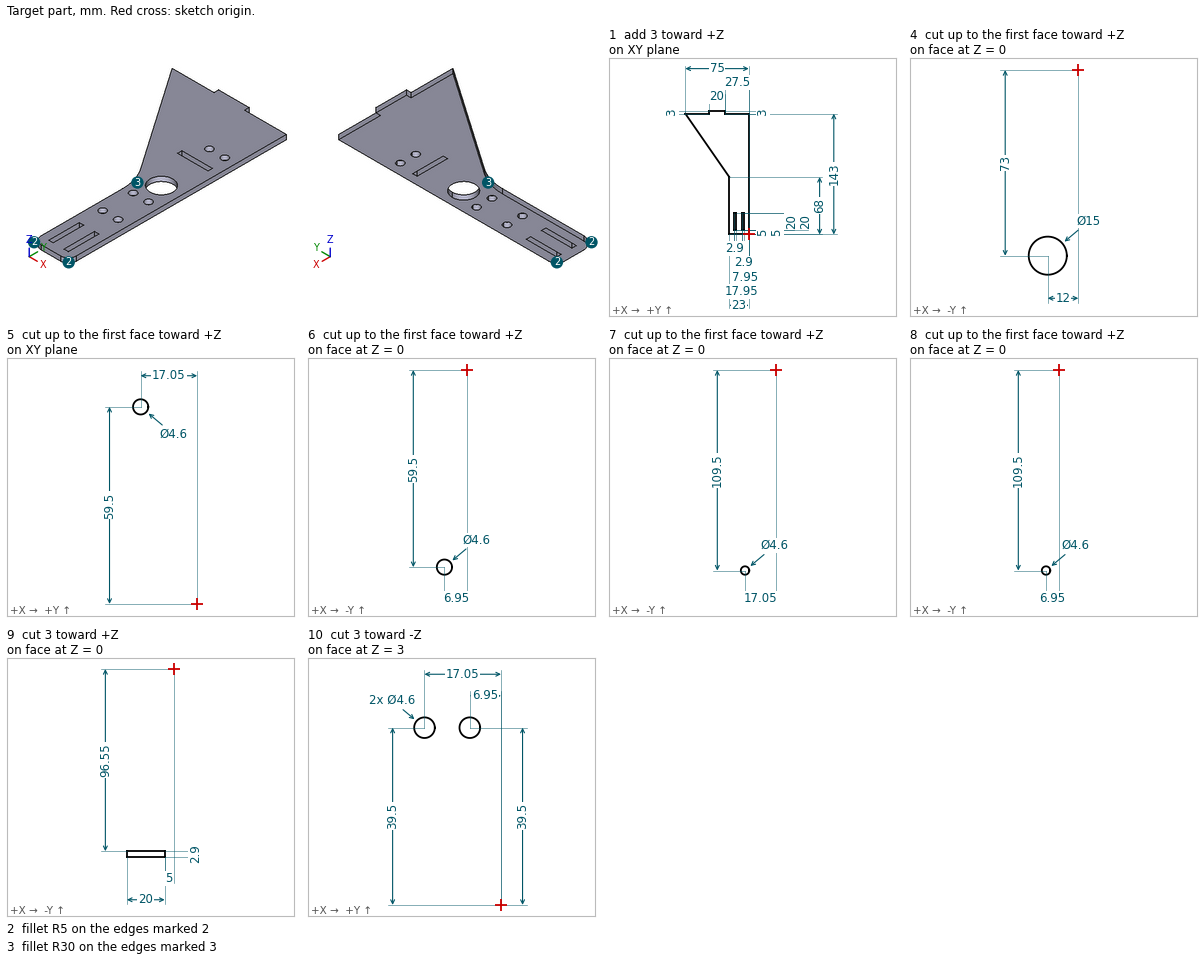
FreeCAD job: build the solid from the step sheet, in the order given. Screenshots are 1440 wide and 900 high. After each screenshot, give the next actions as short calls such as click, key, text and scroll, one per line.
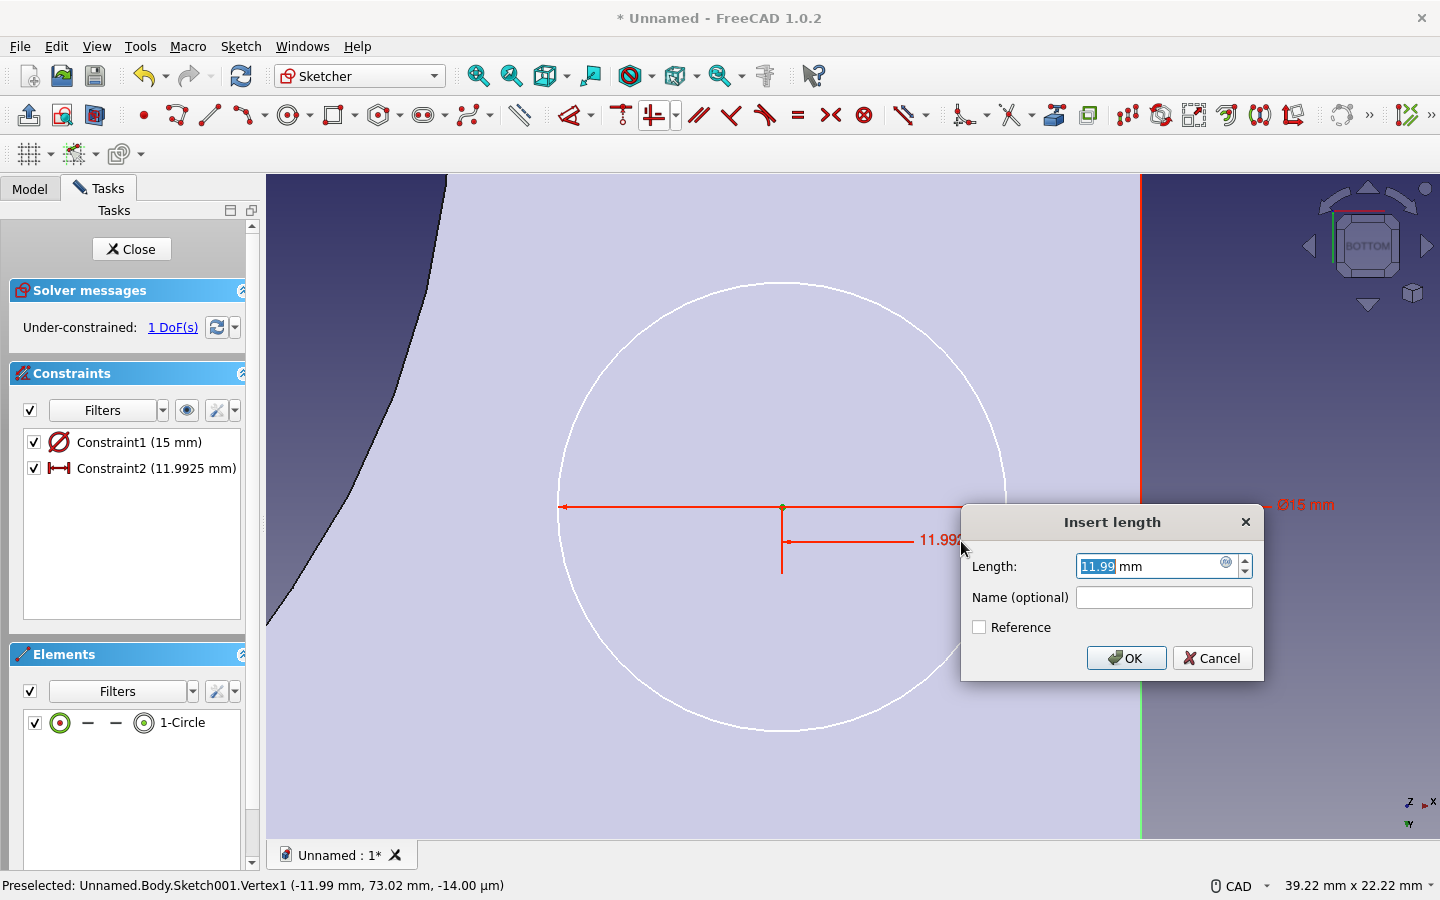
text(12)
key(Return)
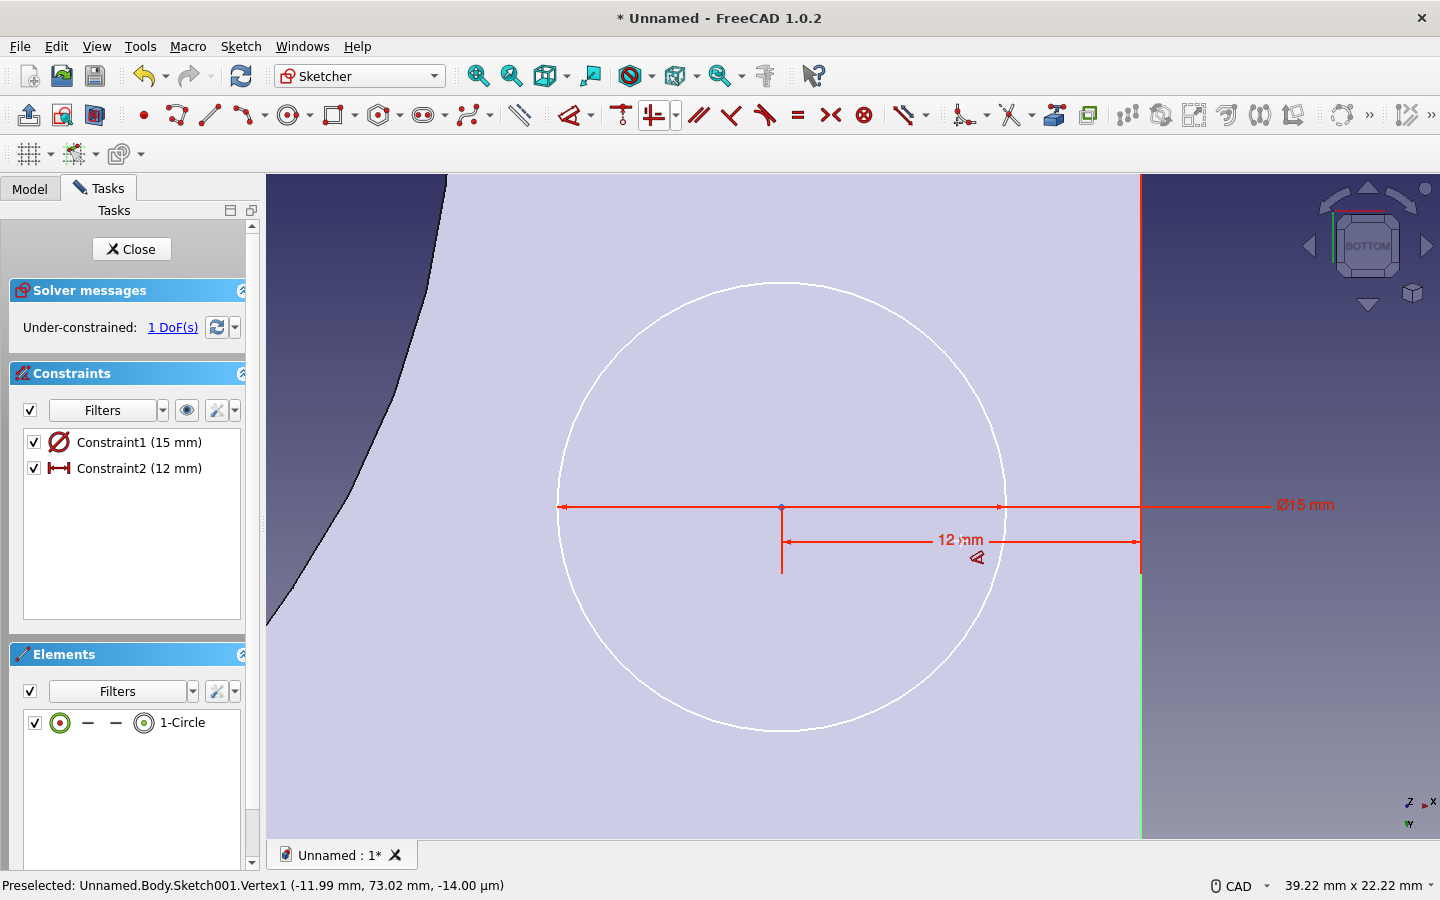
click(782, 507)
click(1175, 355)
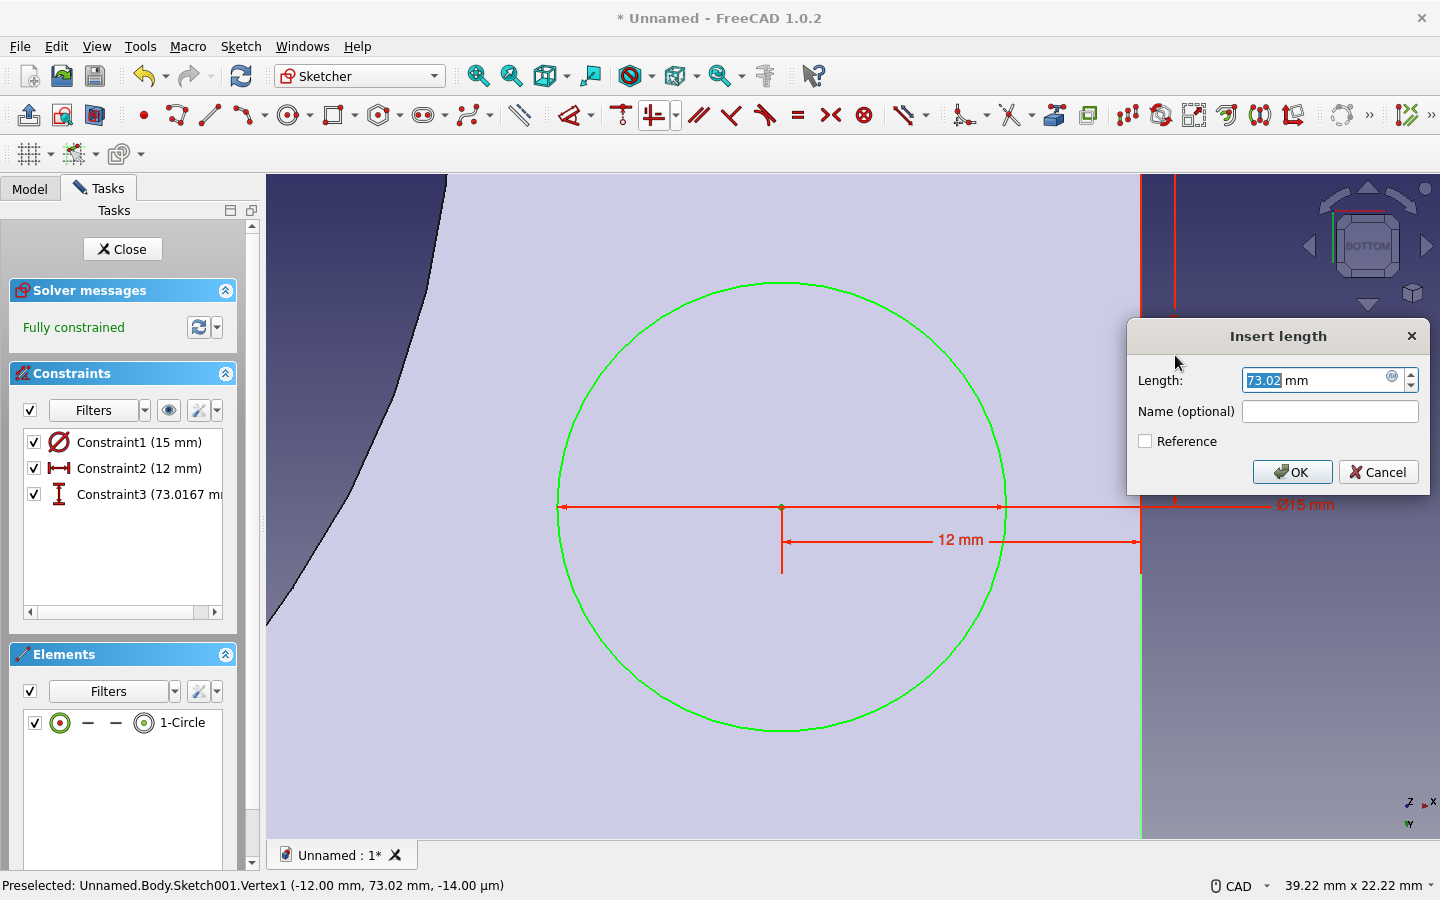
text(73)
key(Return)
key(Escape)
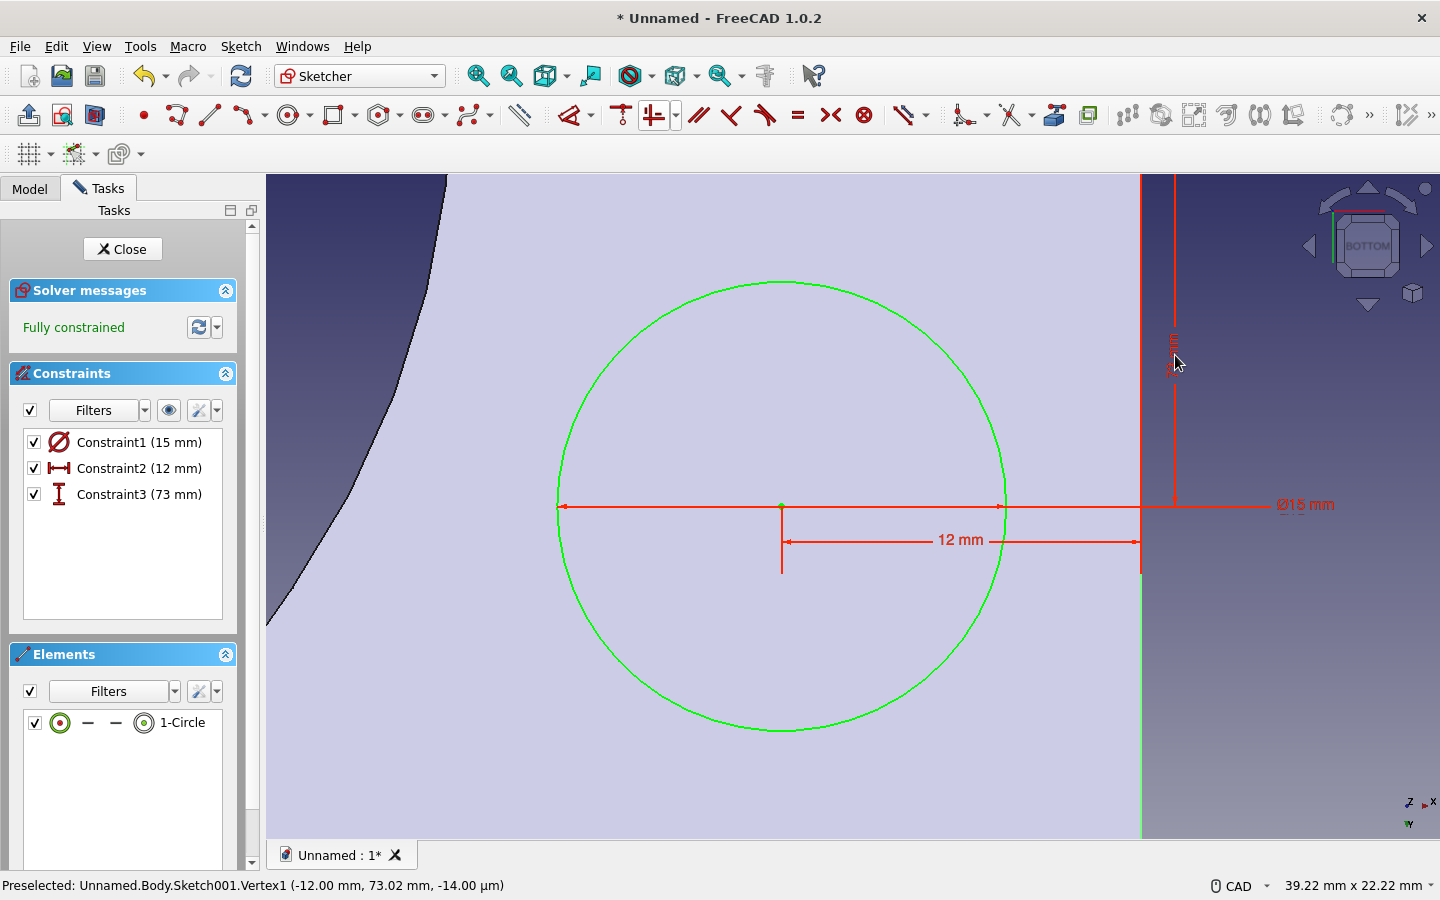
click(123, 249)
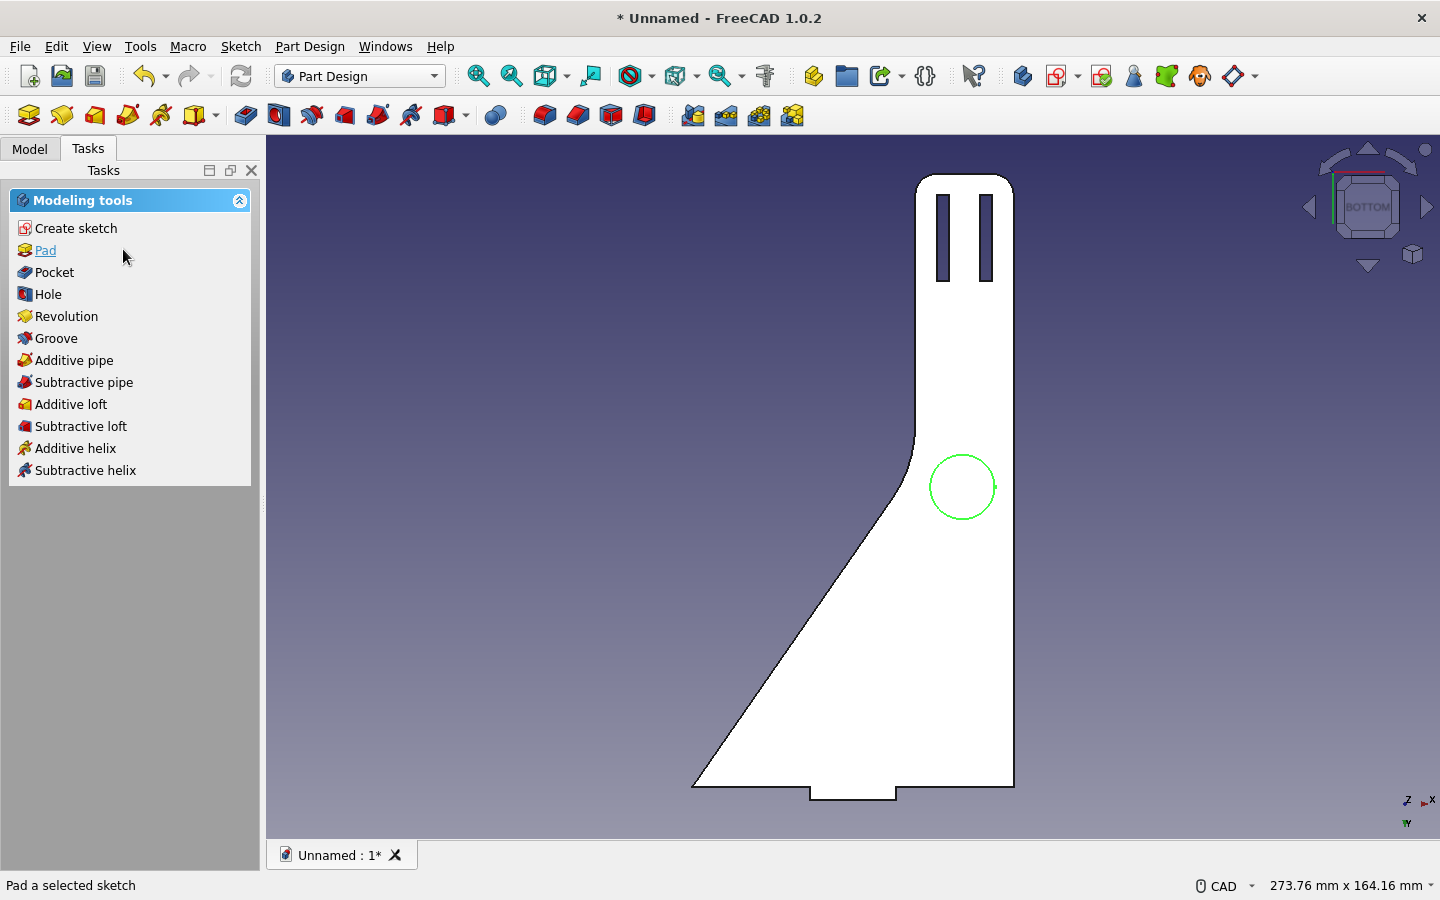
click(246, 116)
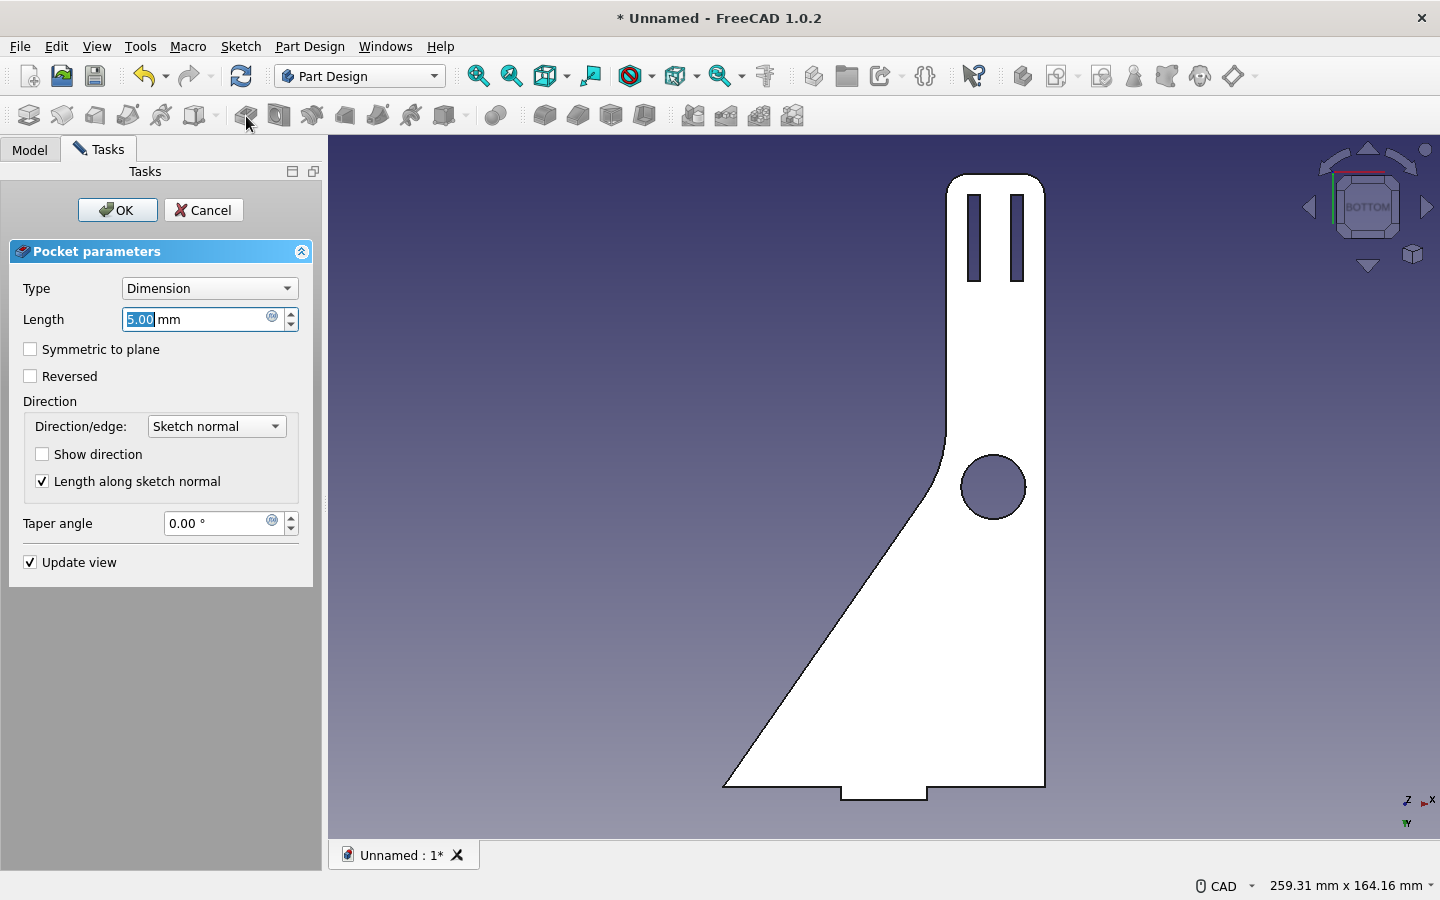
click(210, 288)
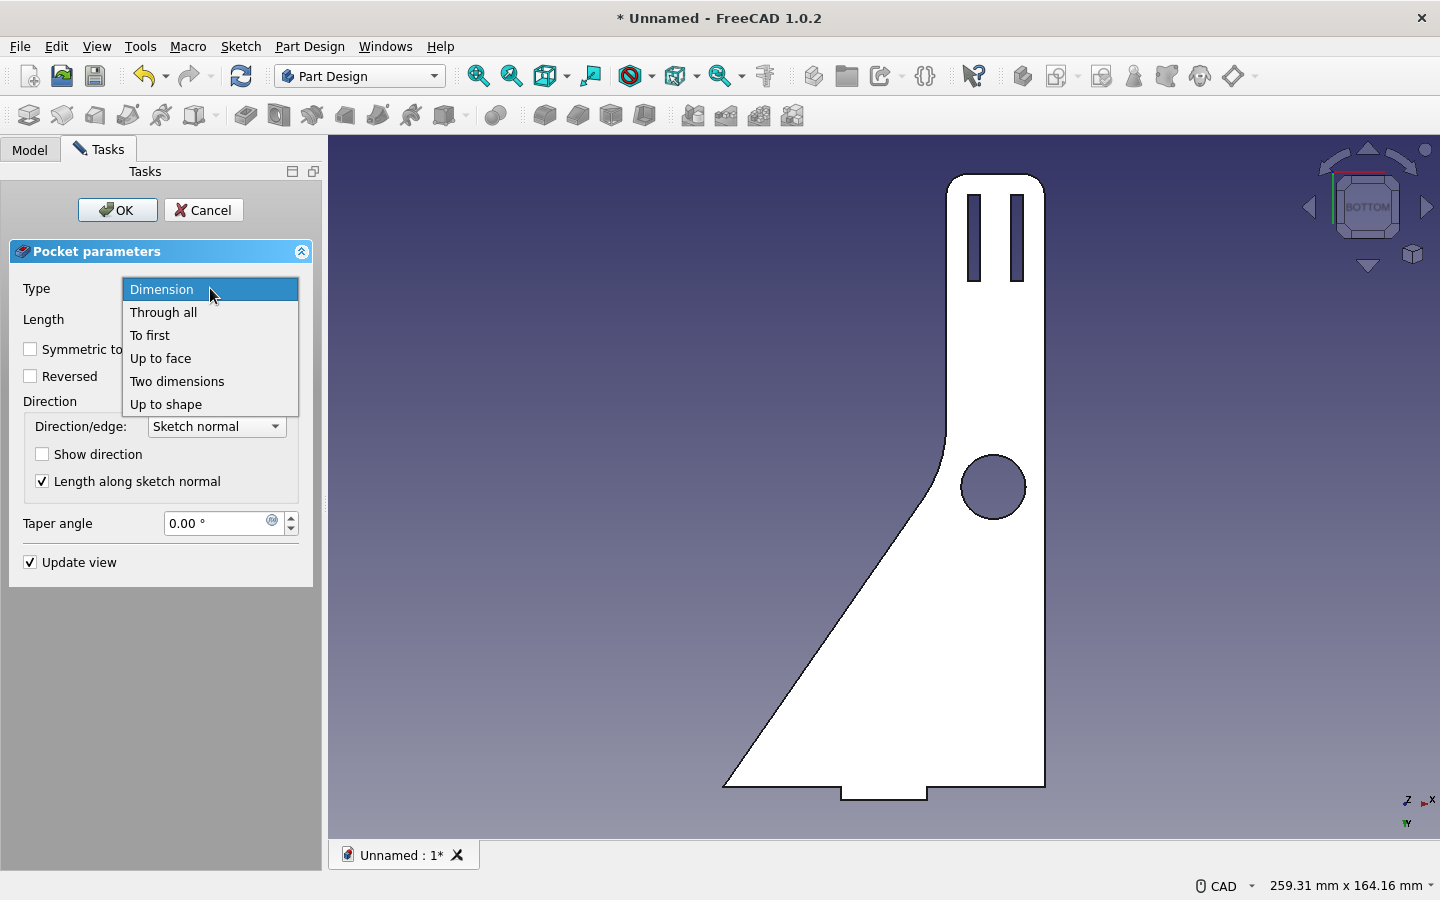
click(208, 336)